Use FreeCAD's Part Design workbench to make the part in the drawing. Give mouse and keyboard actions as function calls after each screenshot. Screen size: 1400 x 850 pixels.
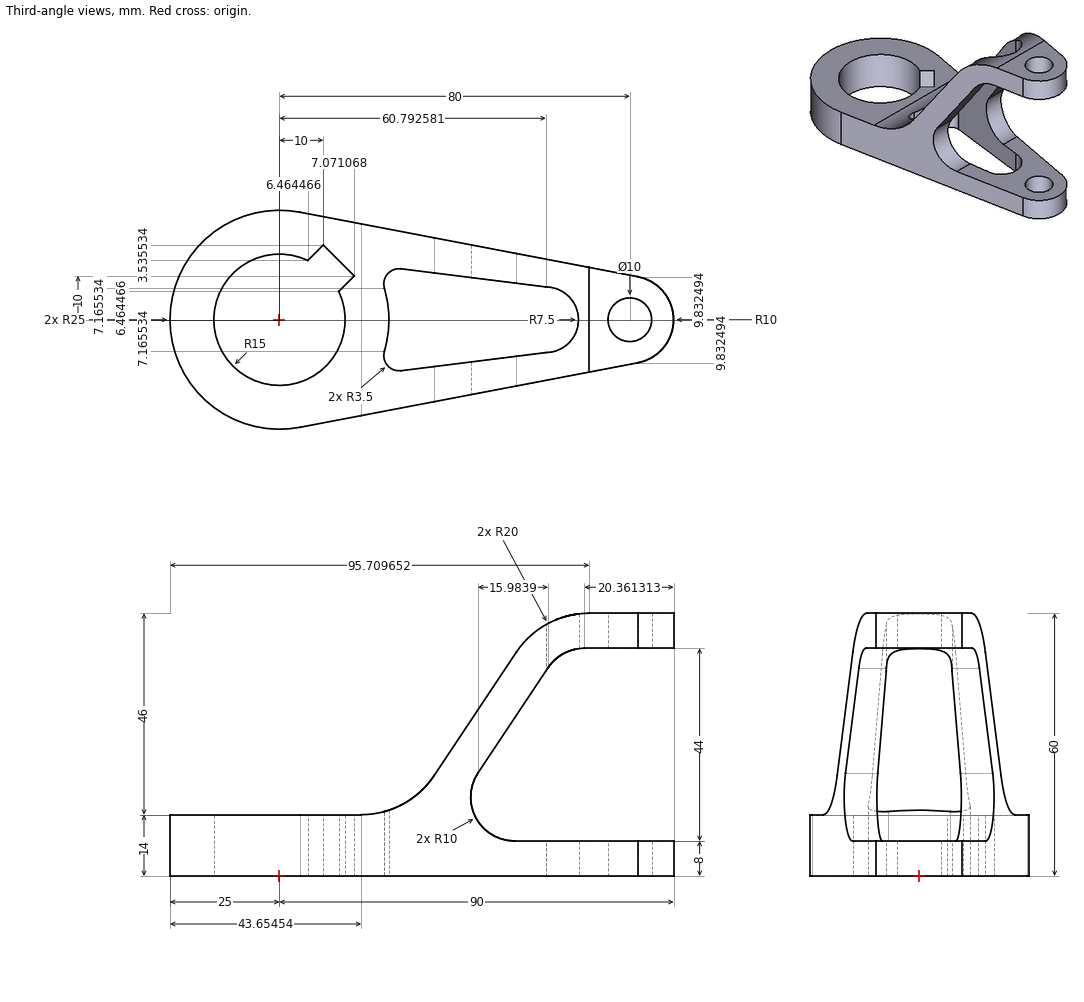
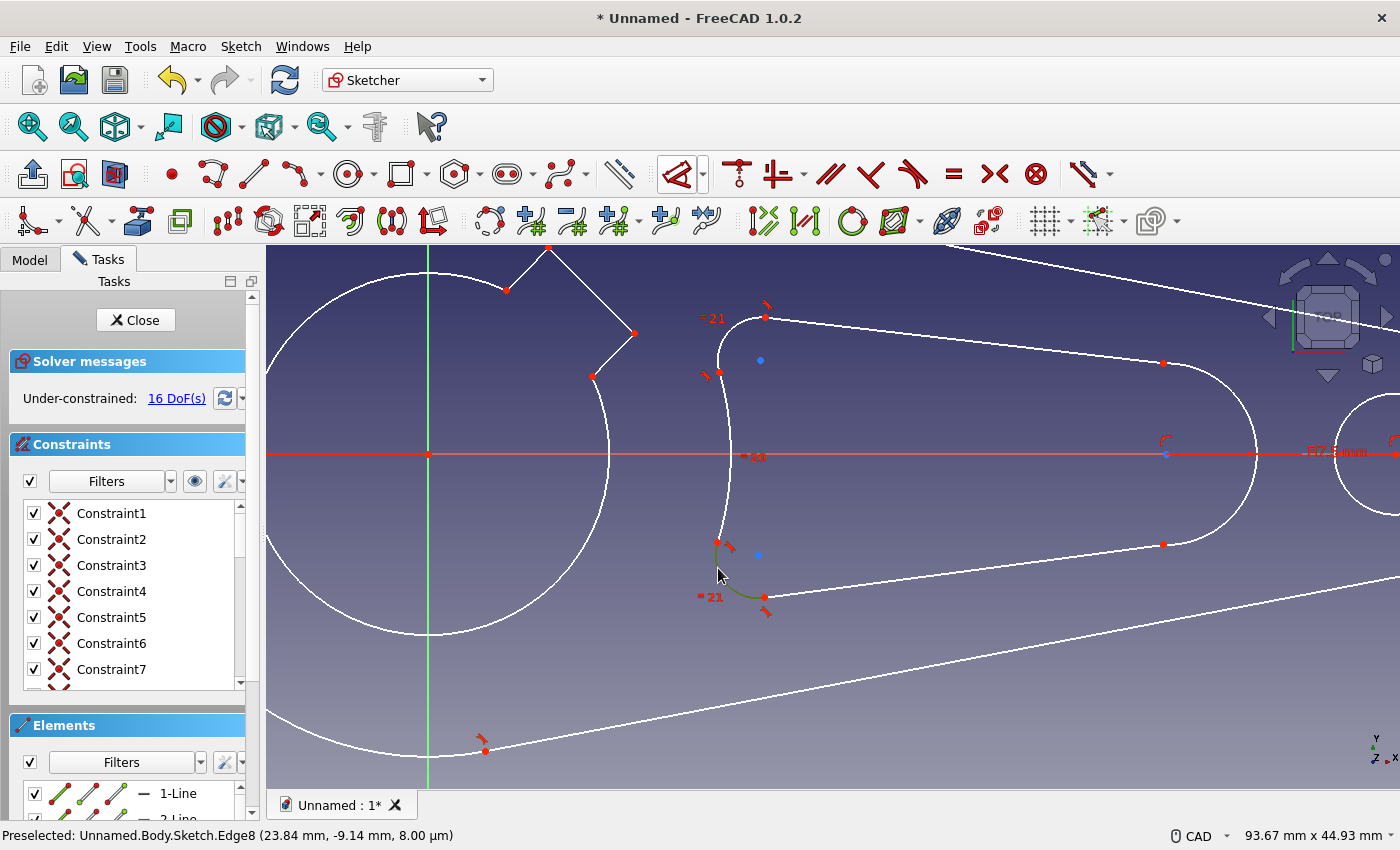
click(702, 174)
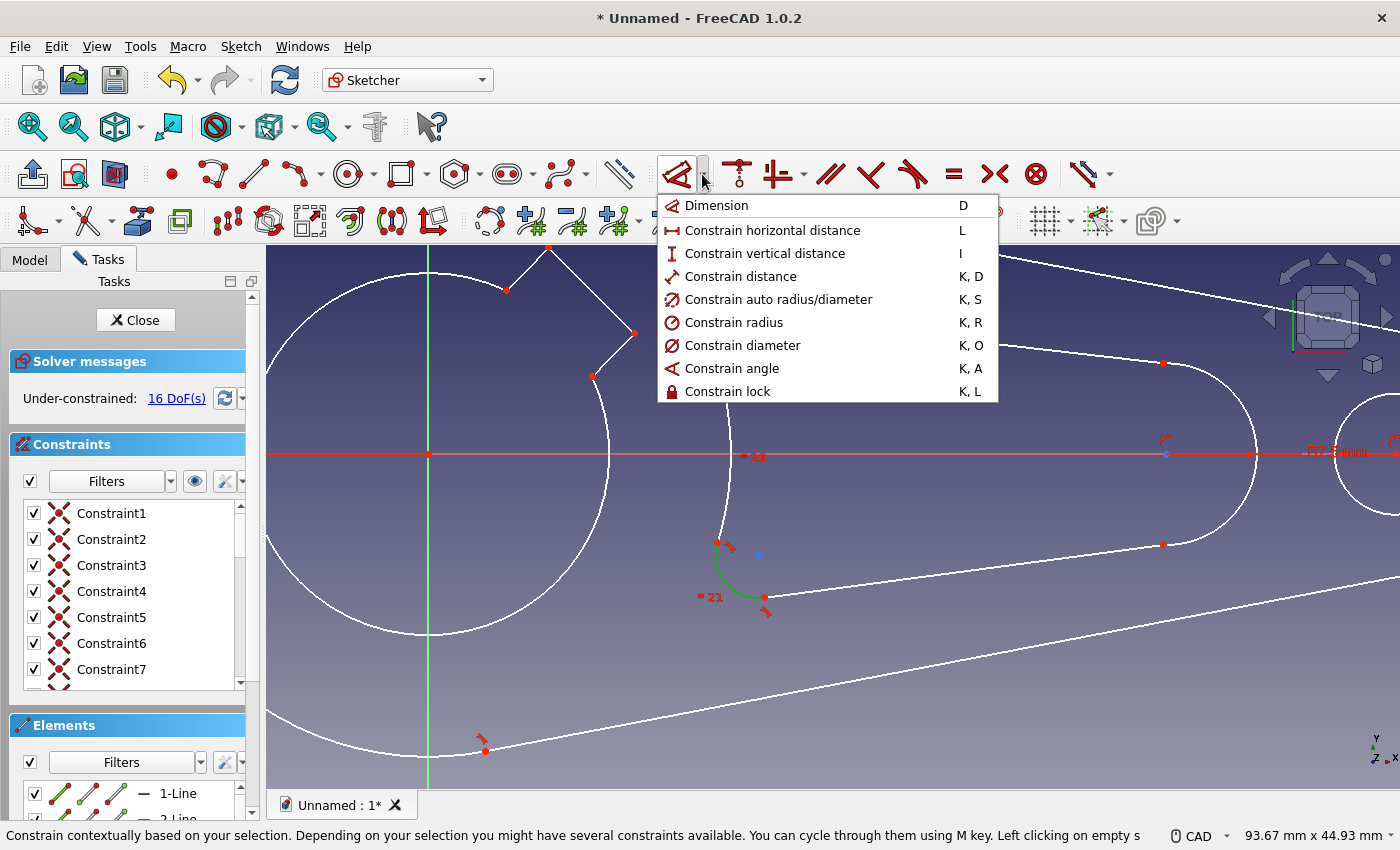
click(828, 322)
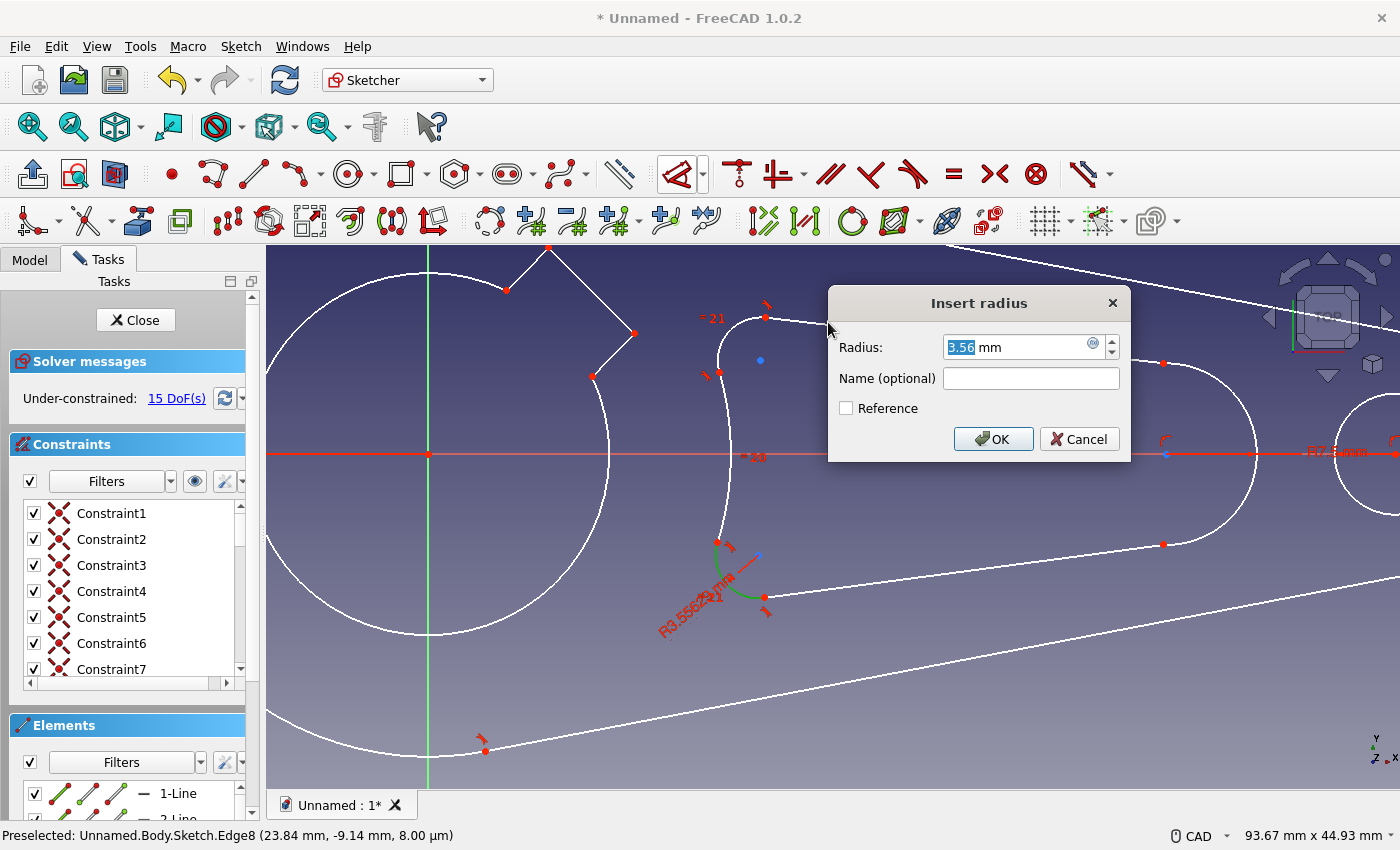
text(3.5)
key(Return)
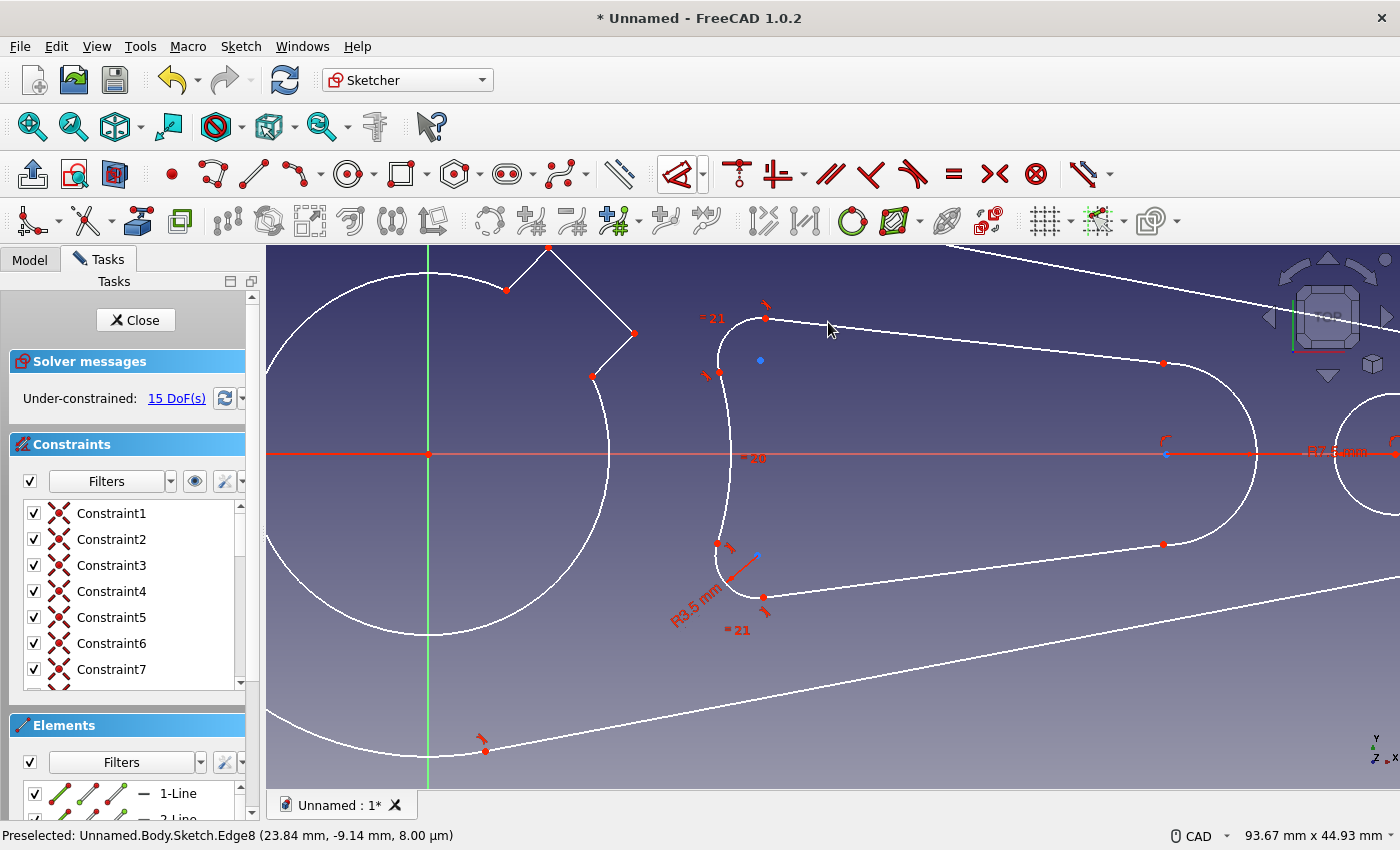
click(487, 625)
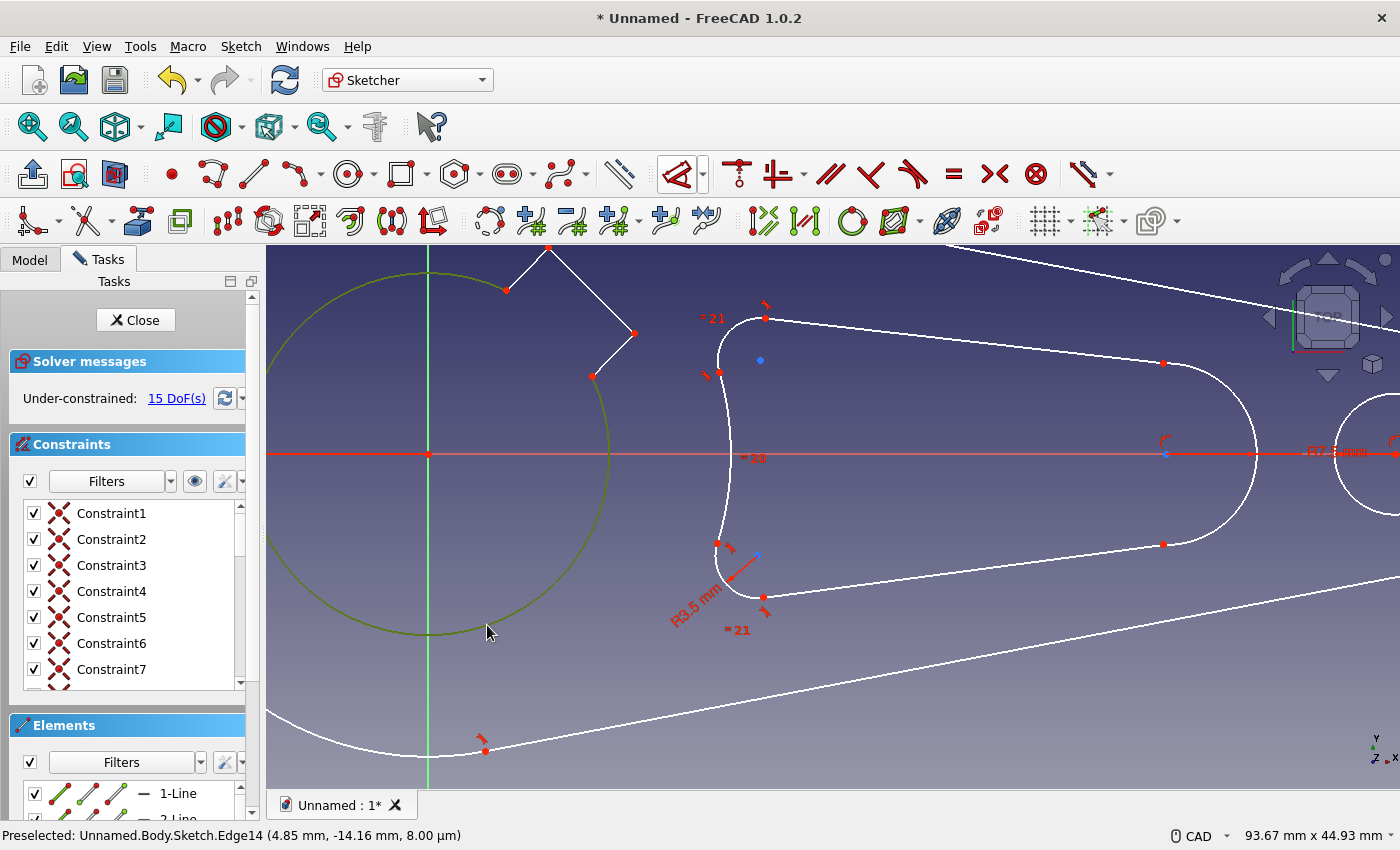
key(k)
key(r)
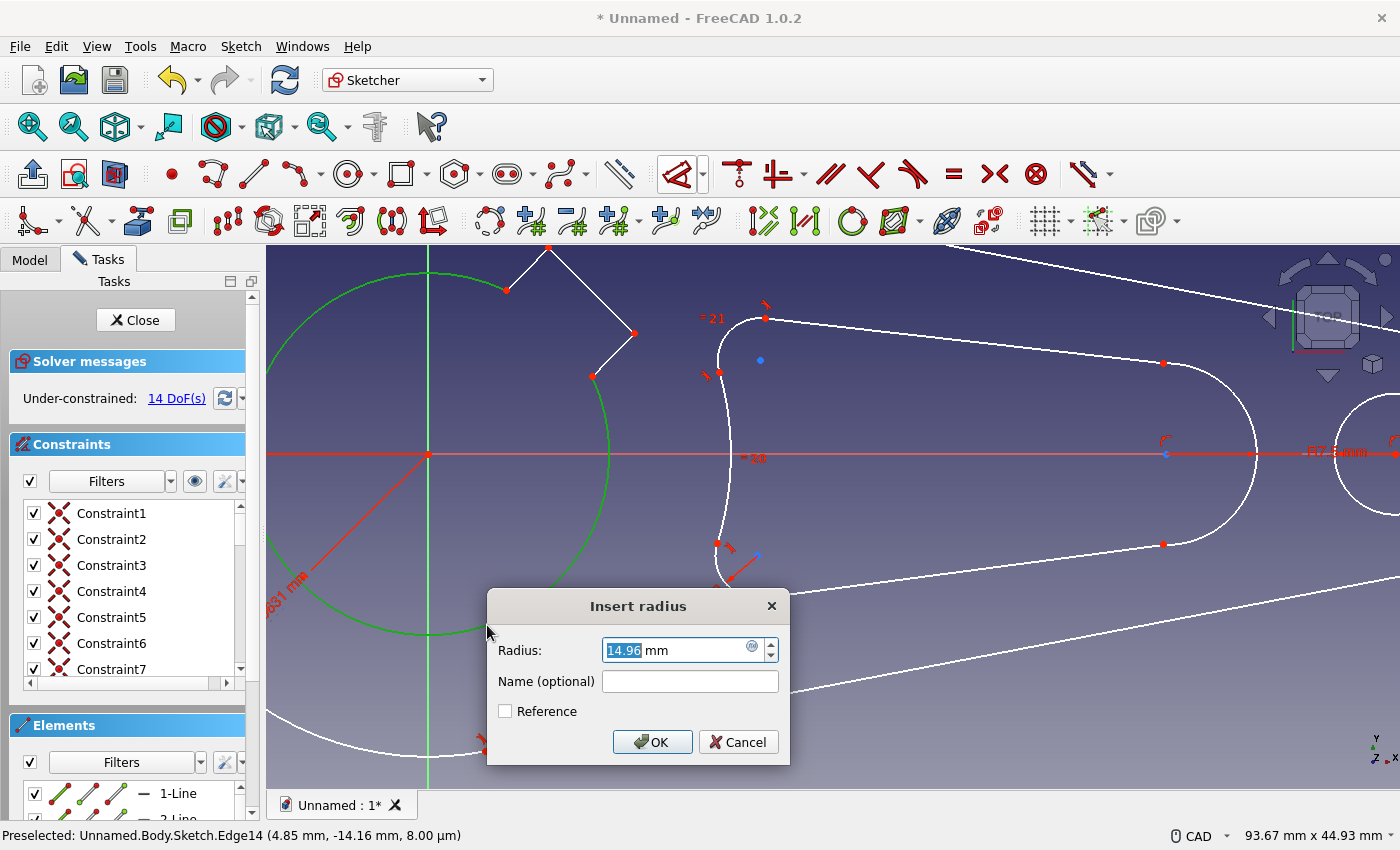
text(15)
key(Return)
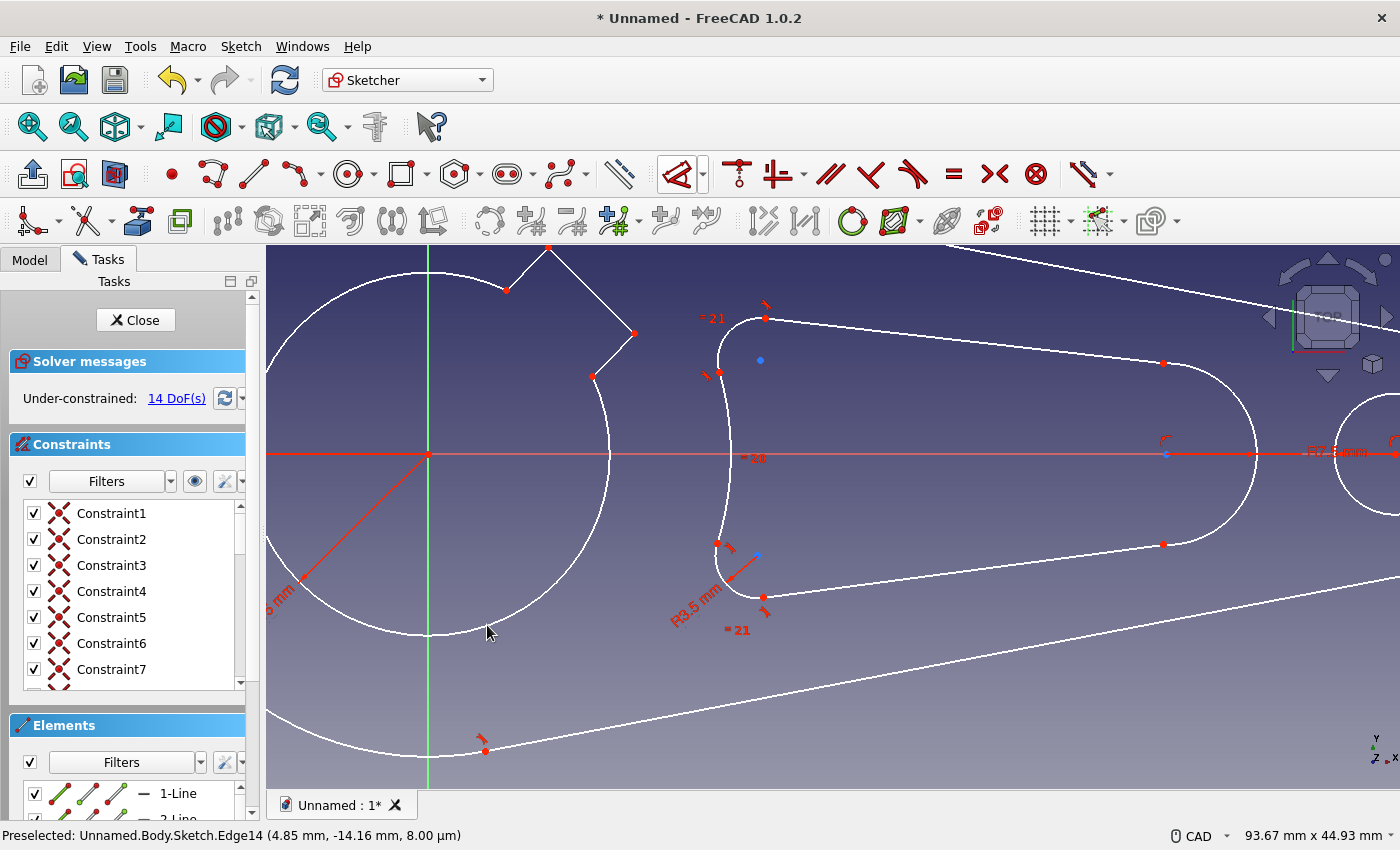
scroll(718, 568, down, 4)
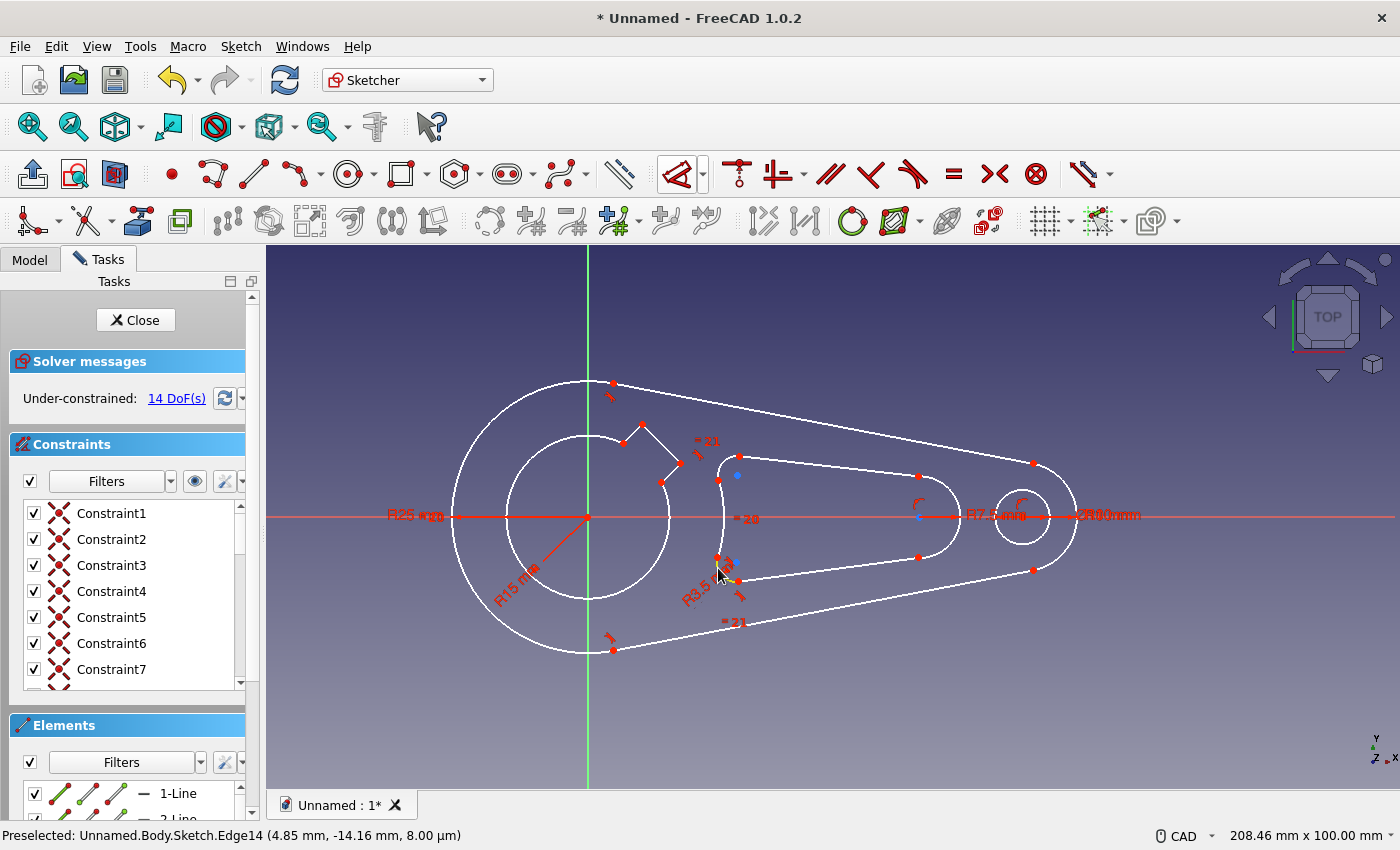
click(1023, 517)